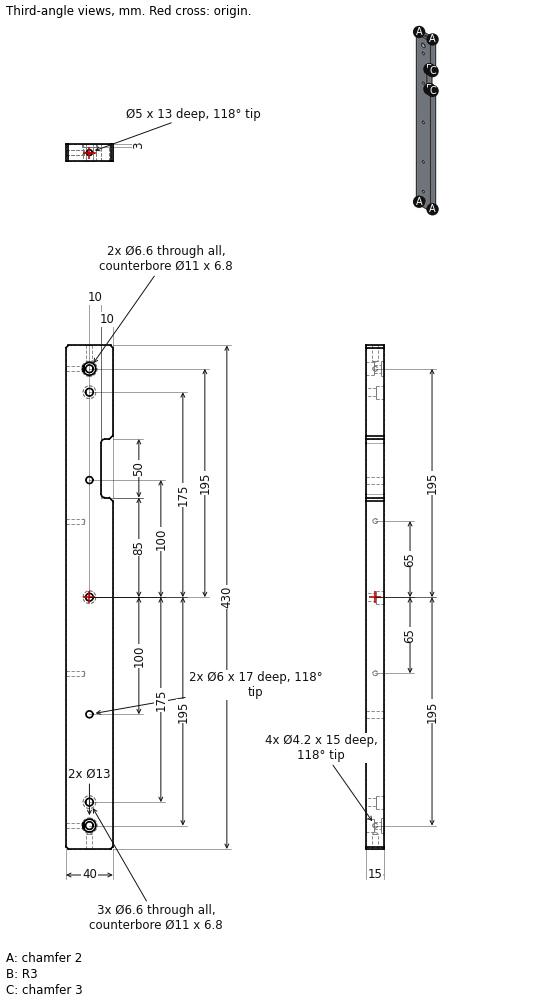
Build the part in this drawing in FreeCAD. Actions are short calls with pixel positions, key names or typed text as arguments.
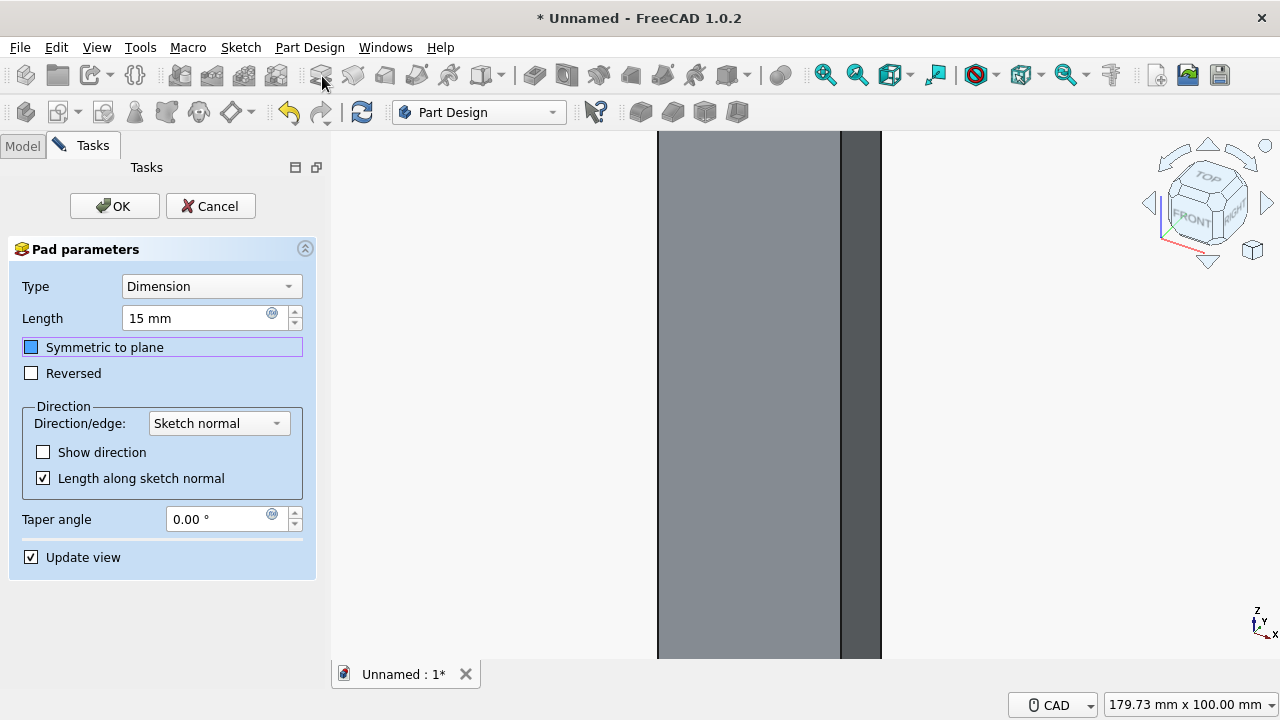
click(30, 347)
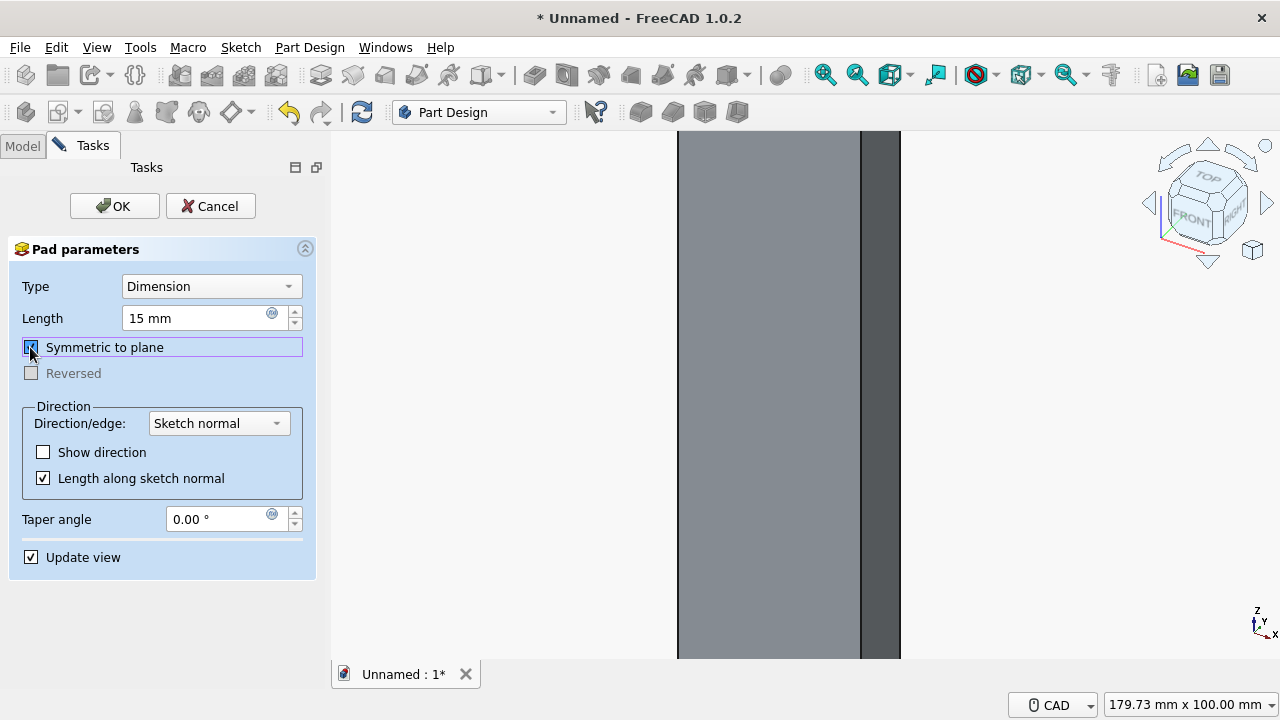
click(115, 206)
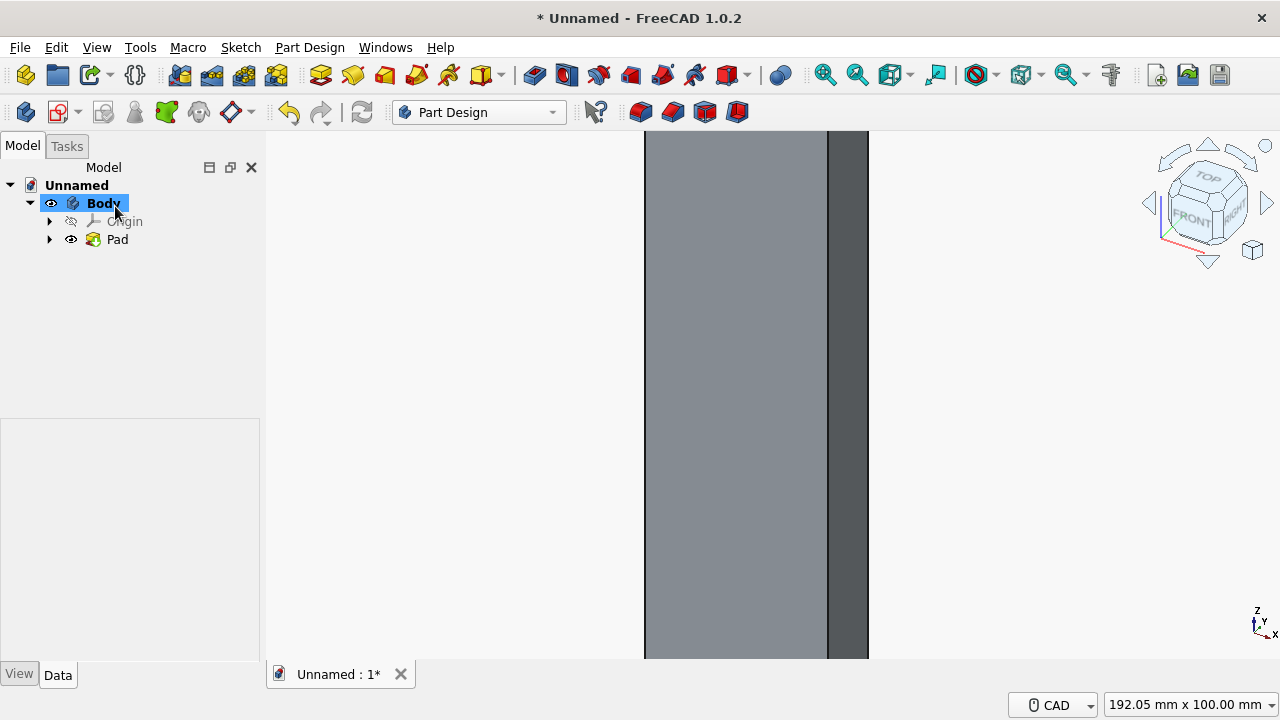
click(826, 76)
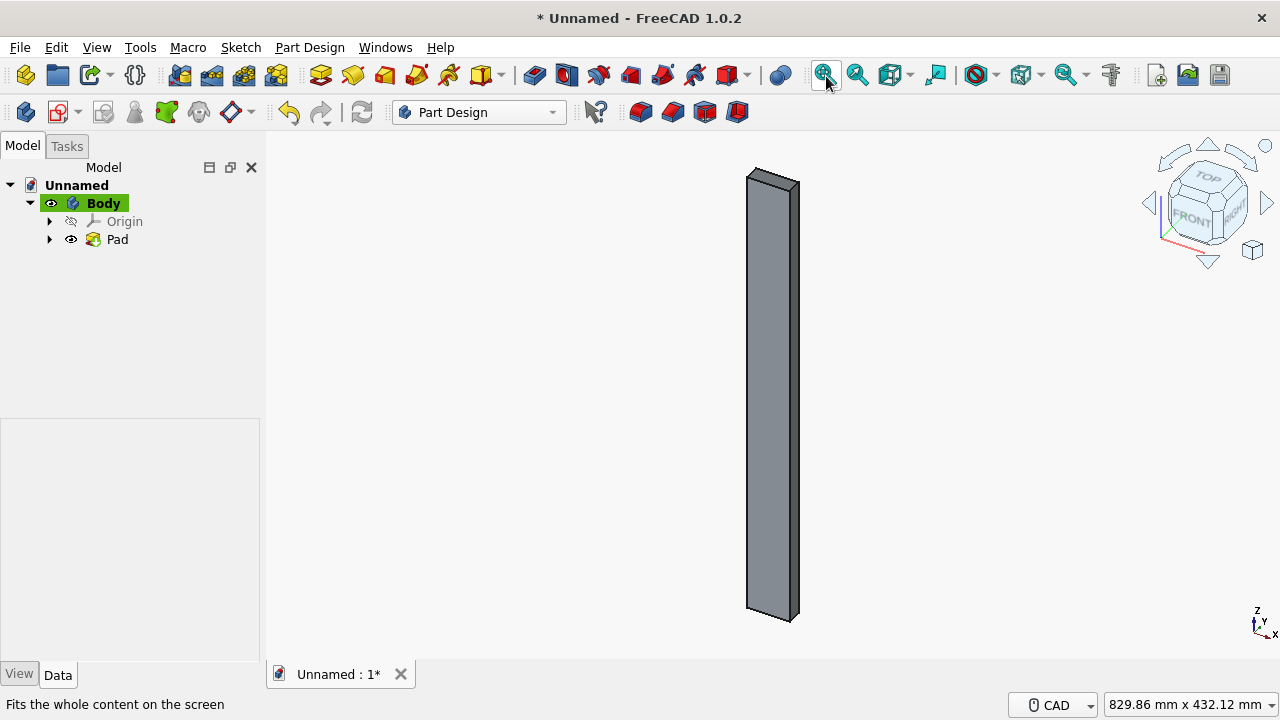
key(4)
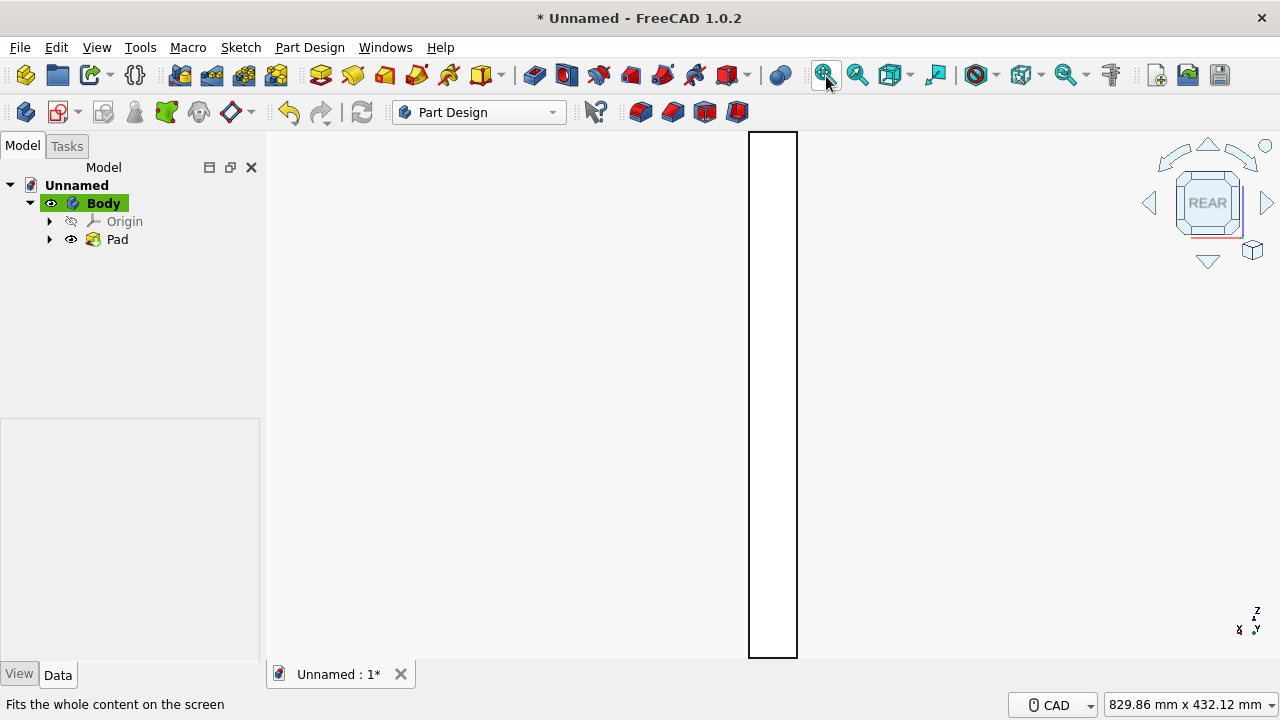
click(773, 169)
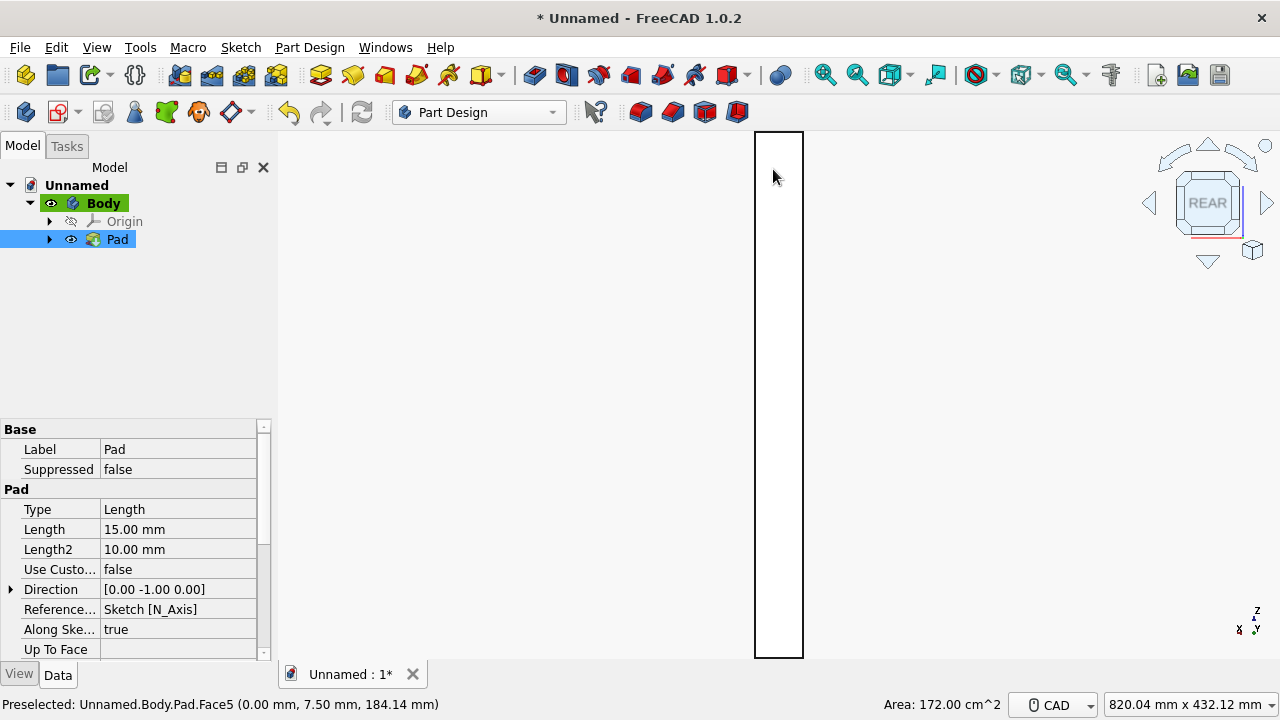
click(58, 112)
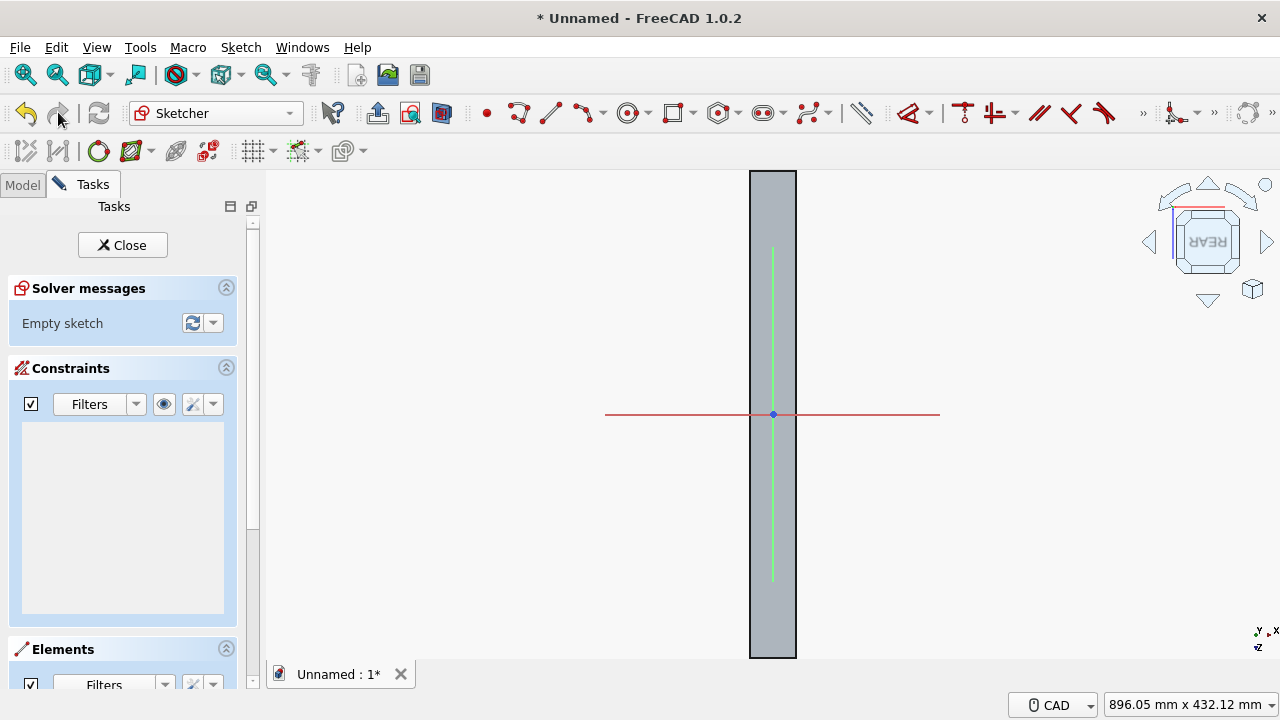
scroll(565, 414, down, 2)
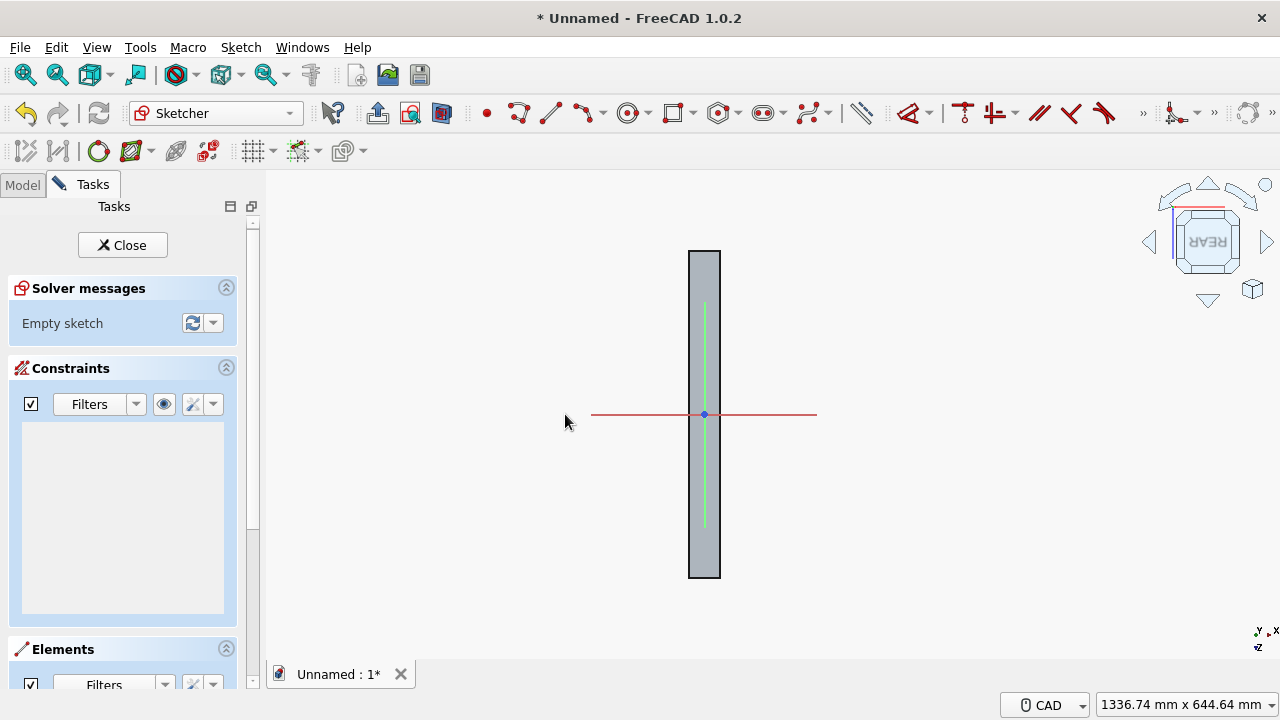
click(628, 114)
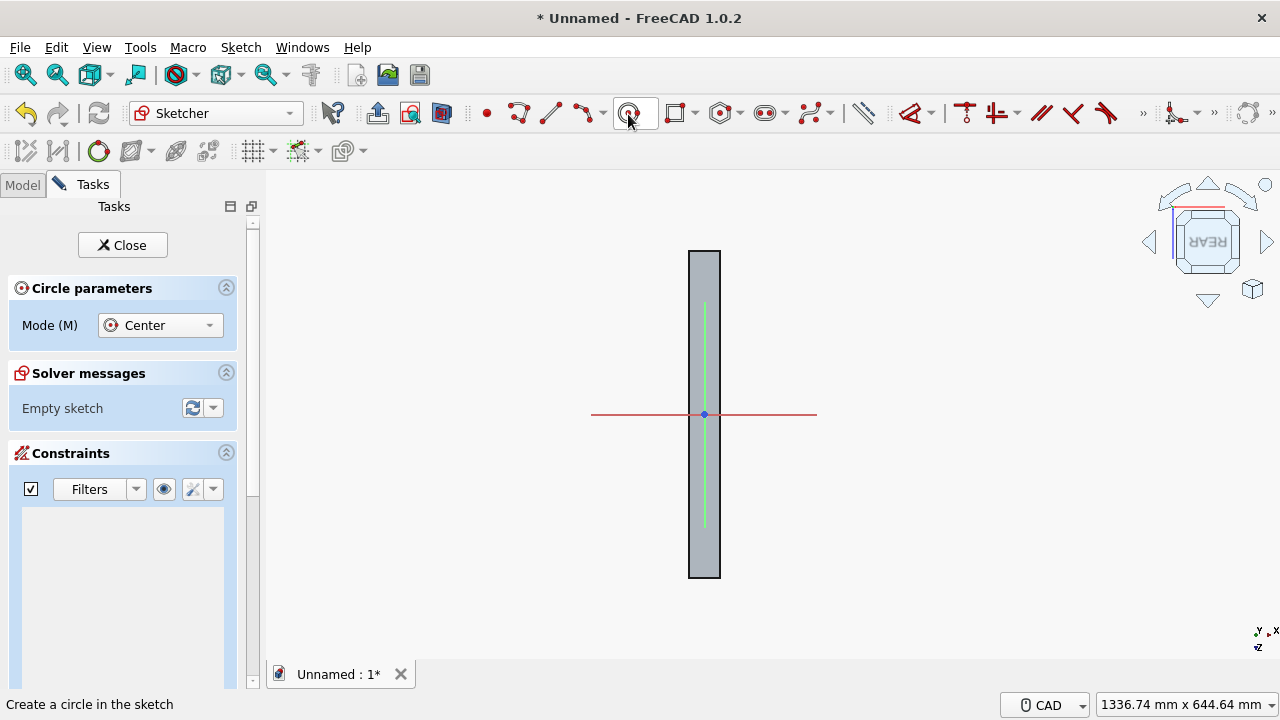
scroll(705, 267, up, 8)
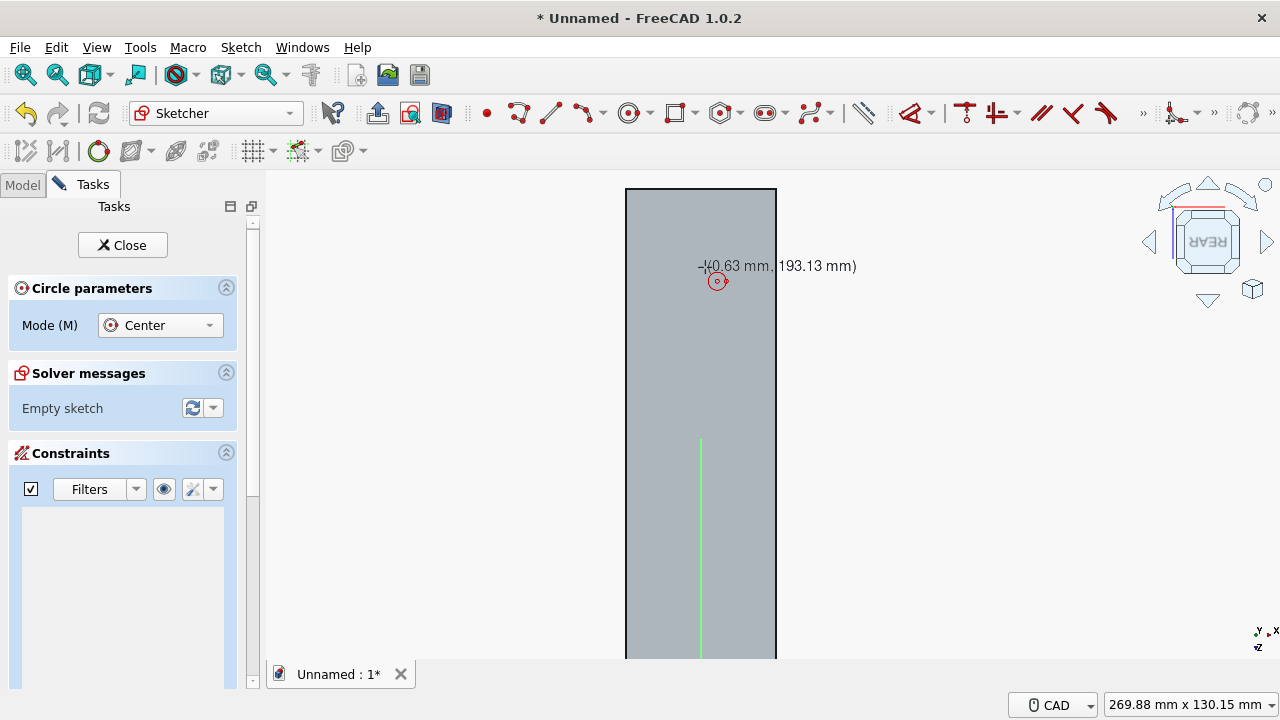
scroll(705, 267, down, 8)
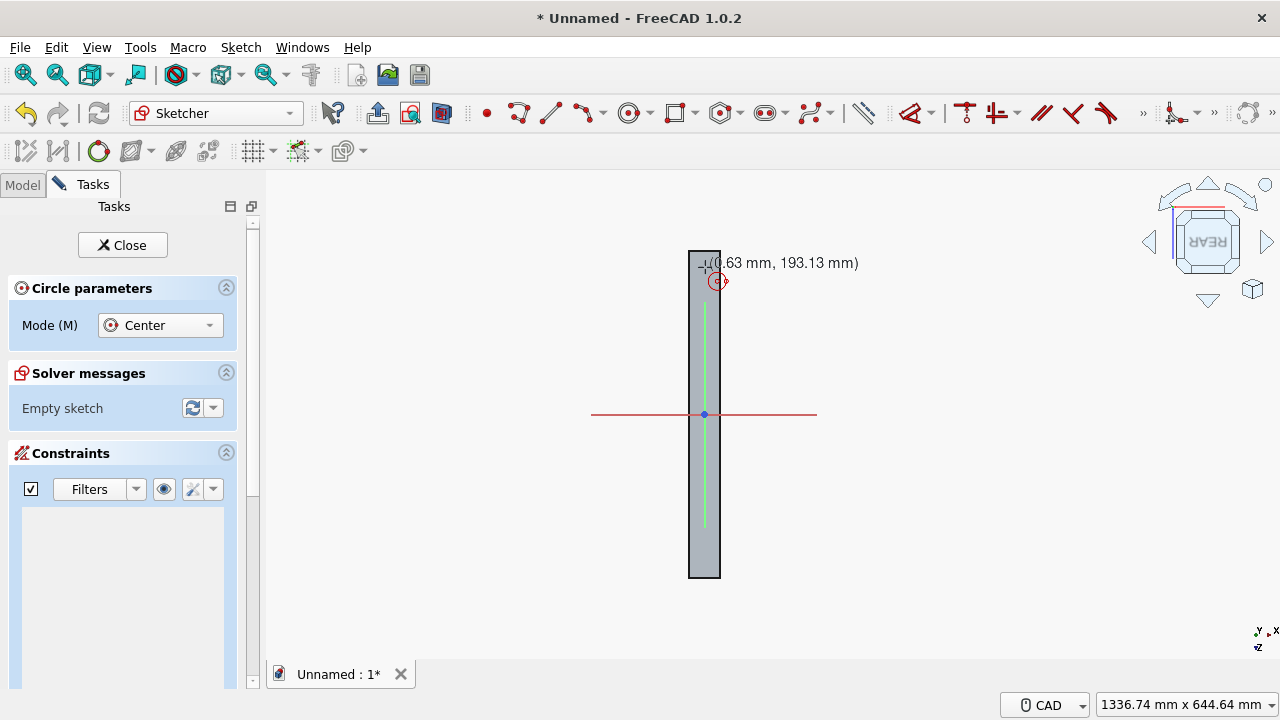
click(705, 267)